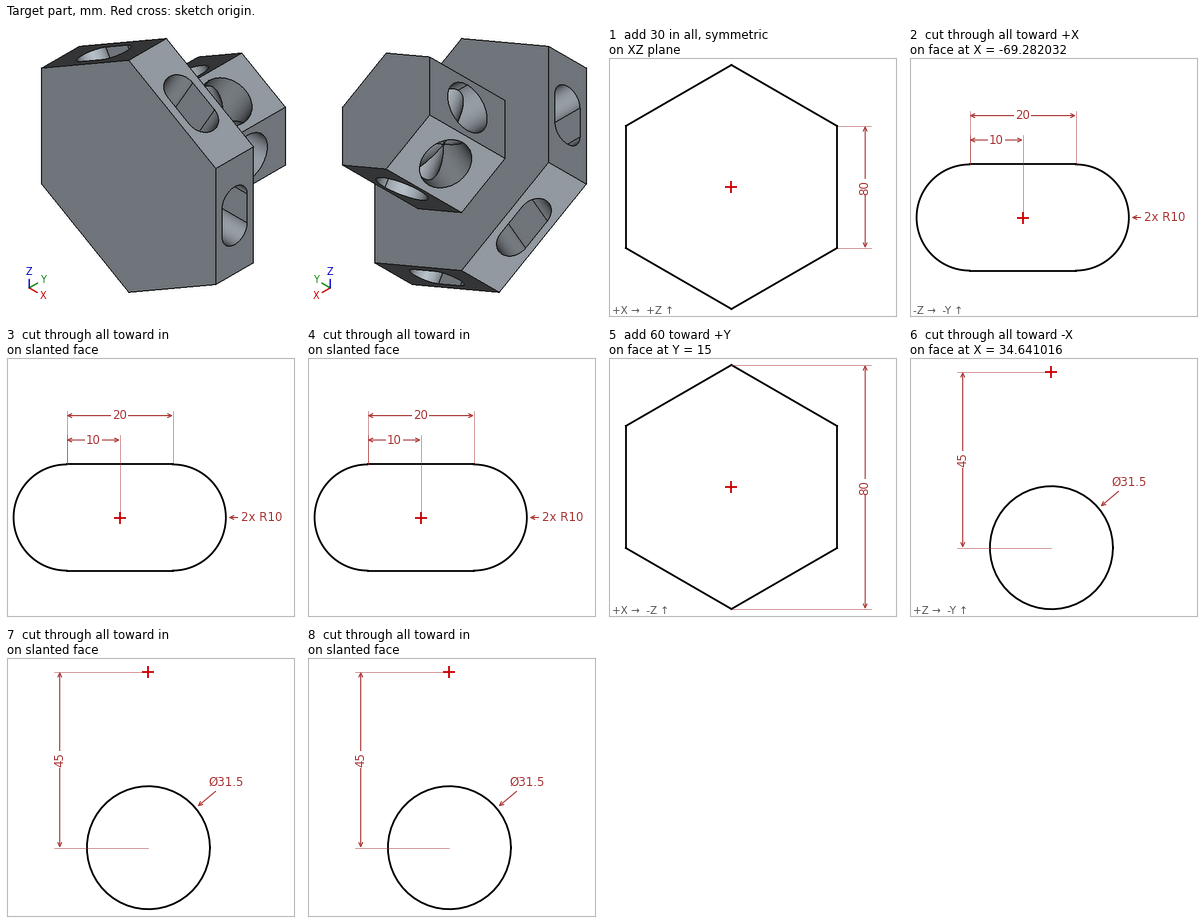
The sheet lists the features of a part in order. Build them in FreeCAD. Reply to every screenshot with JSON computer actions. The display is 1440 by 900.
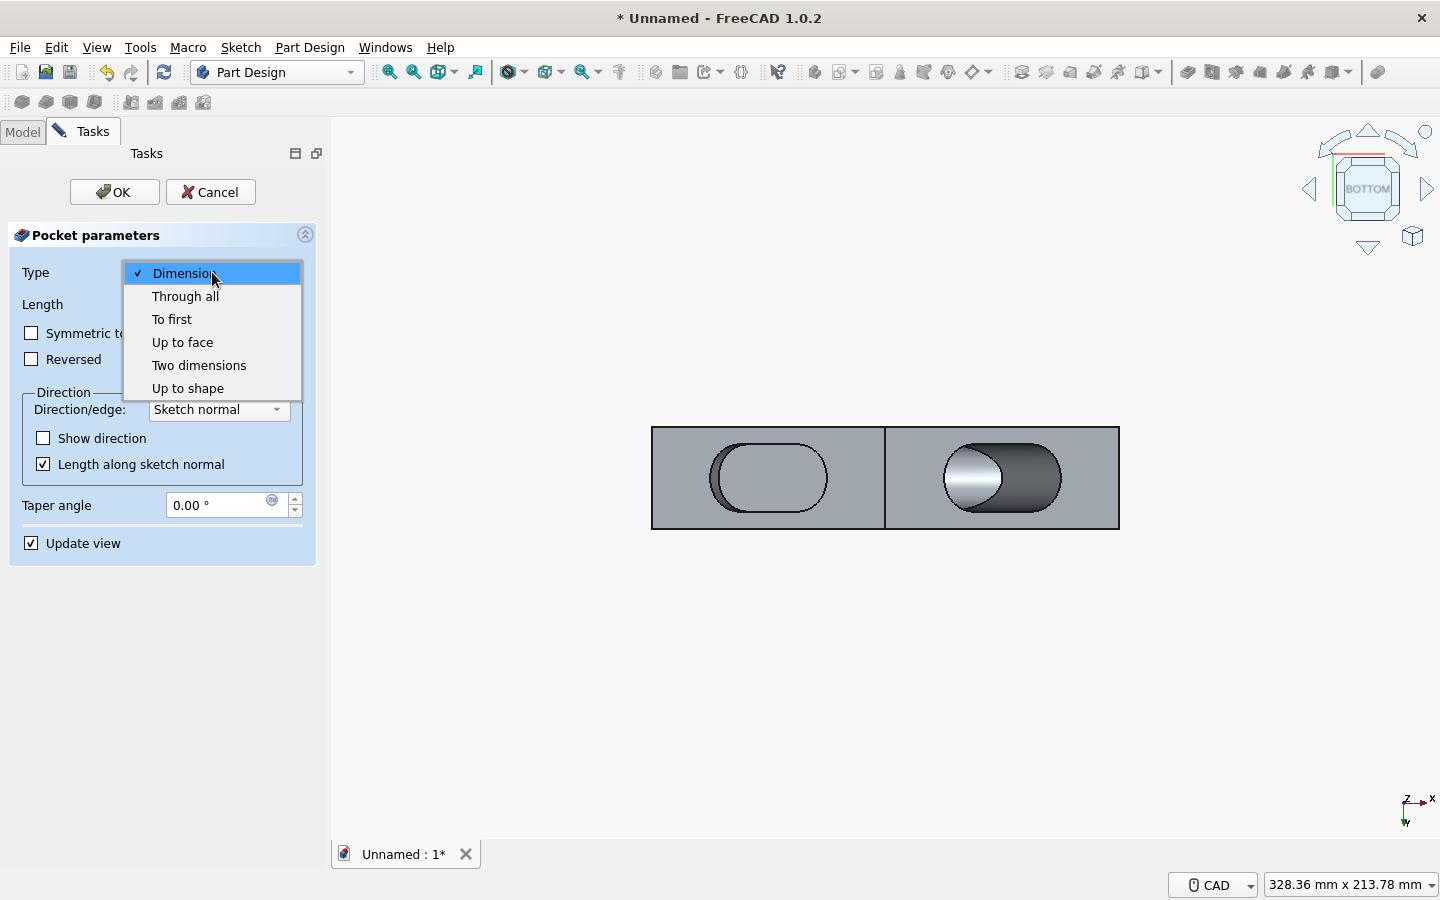
{"action": "left_click", "coordinate": [212, 296]}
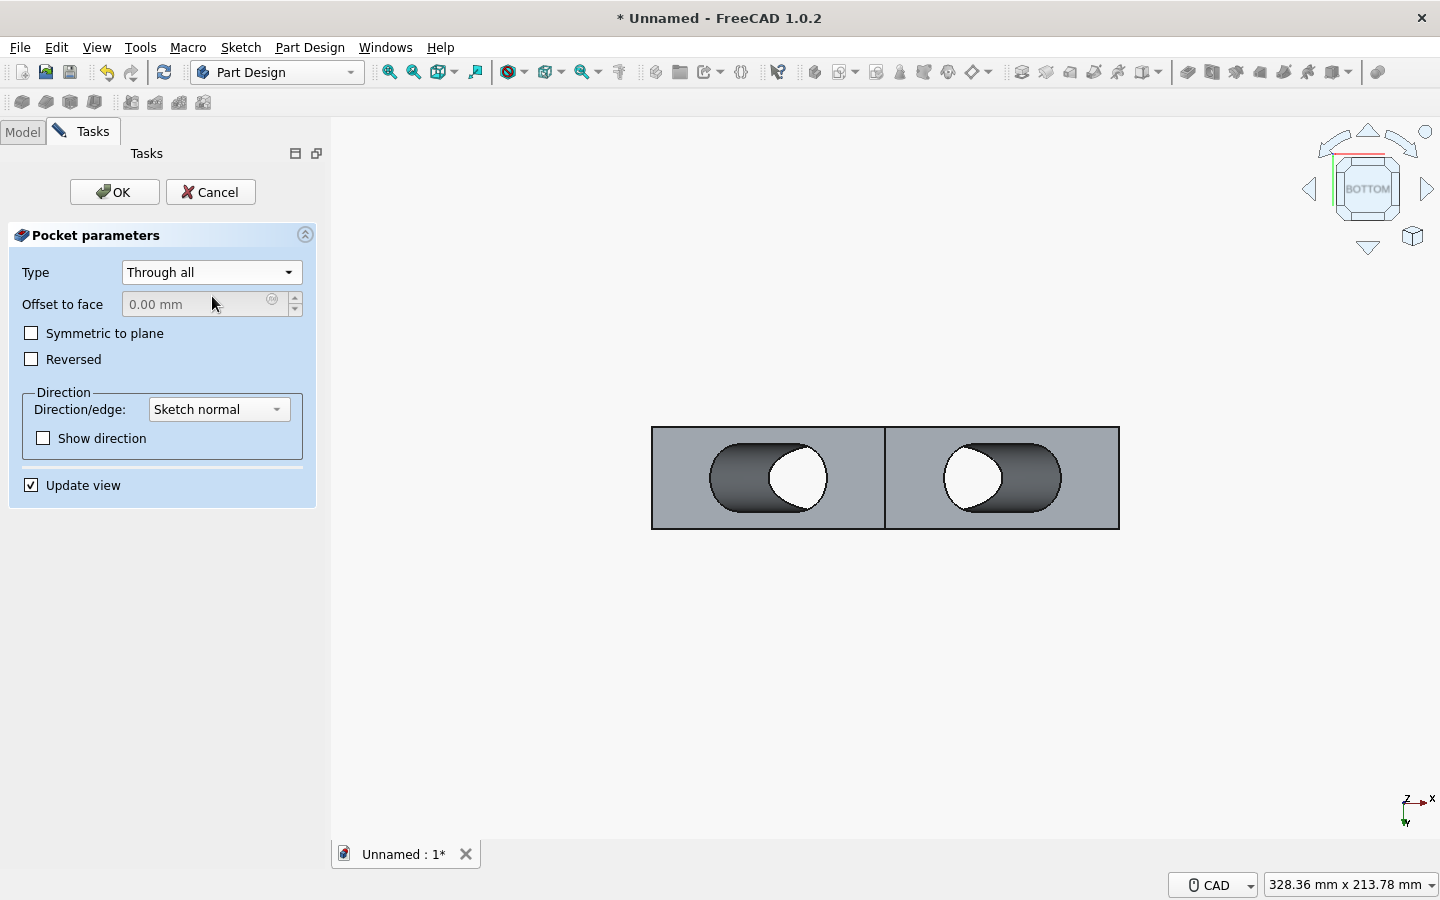
{"action": "left_click", "coordinate": [115, 192]}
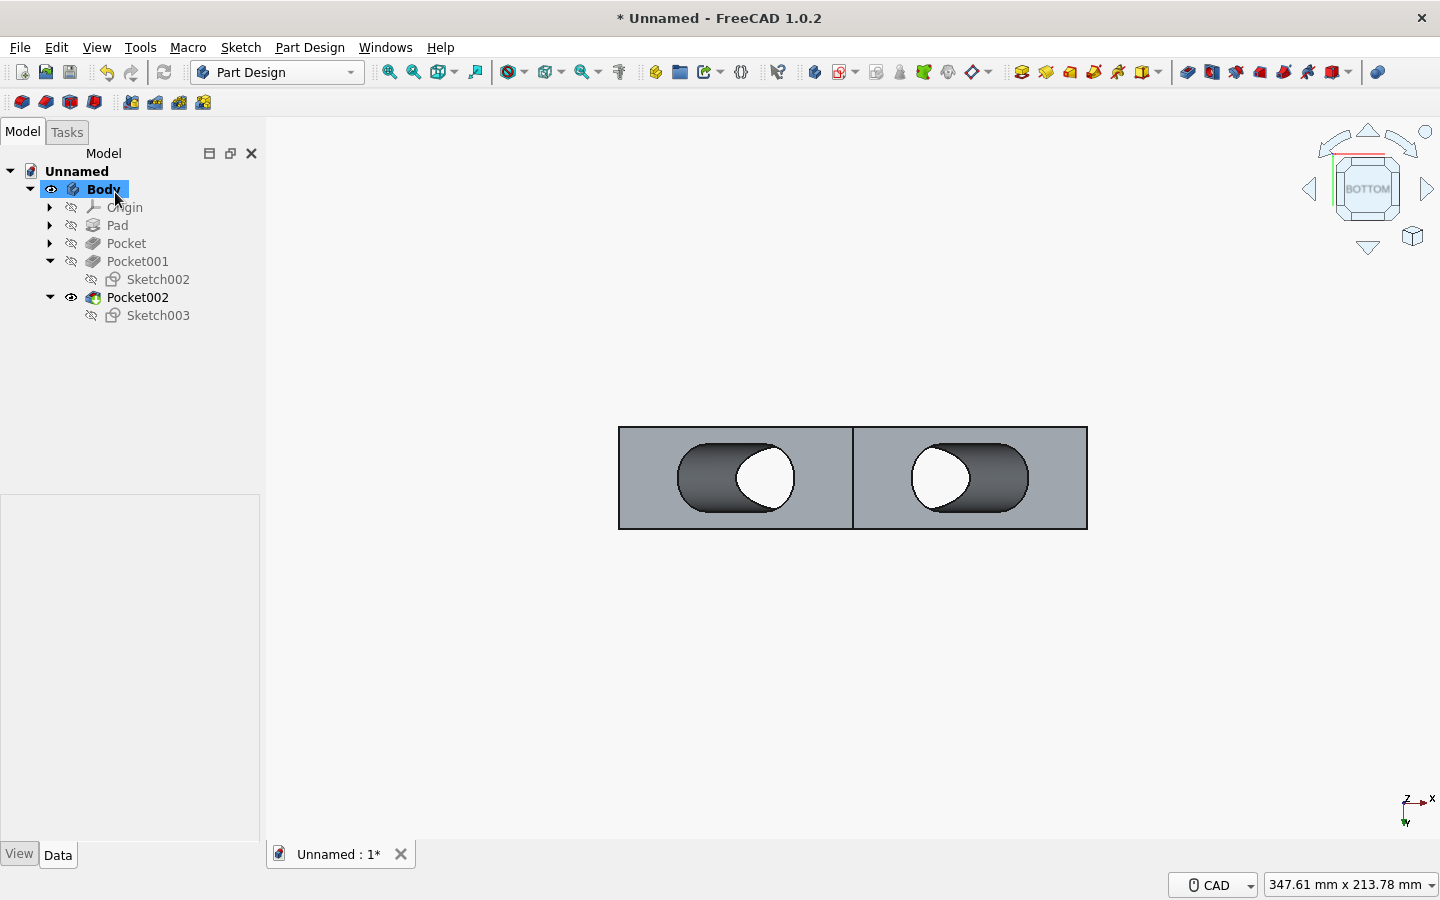
{"action": "left_click", "coordinate": [390, 72]}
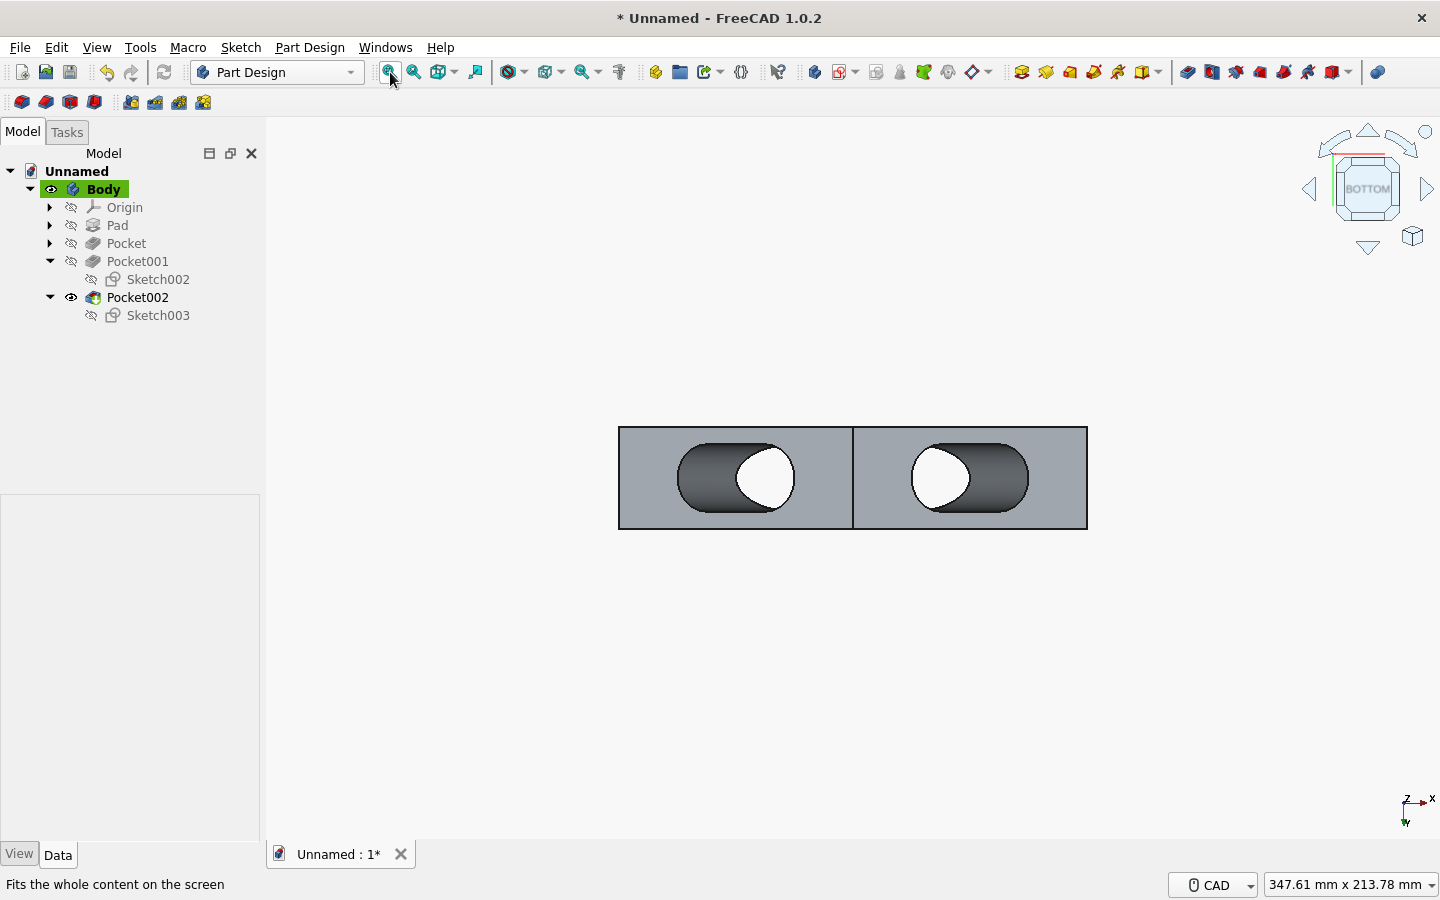
{"action": "key", "text": "4"}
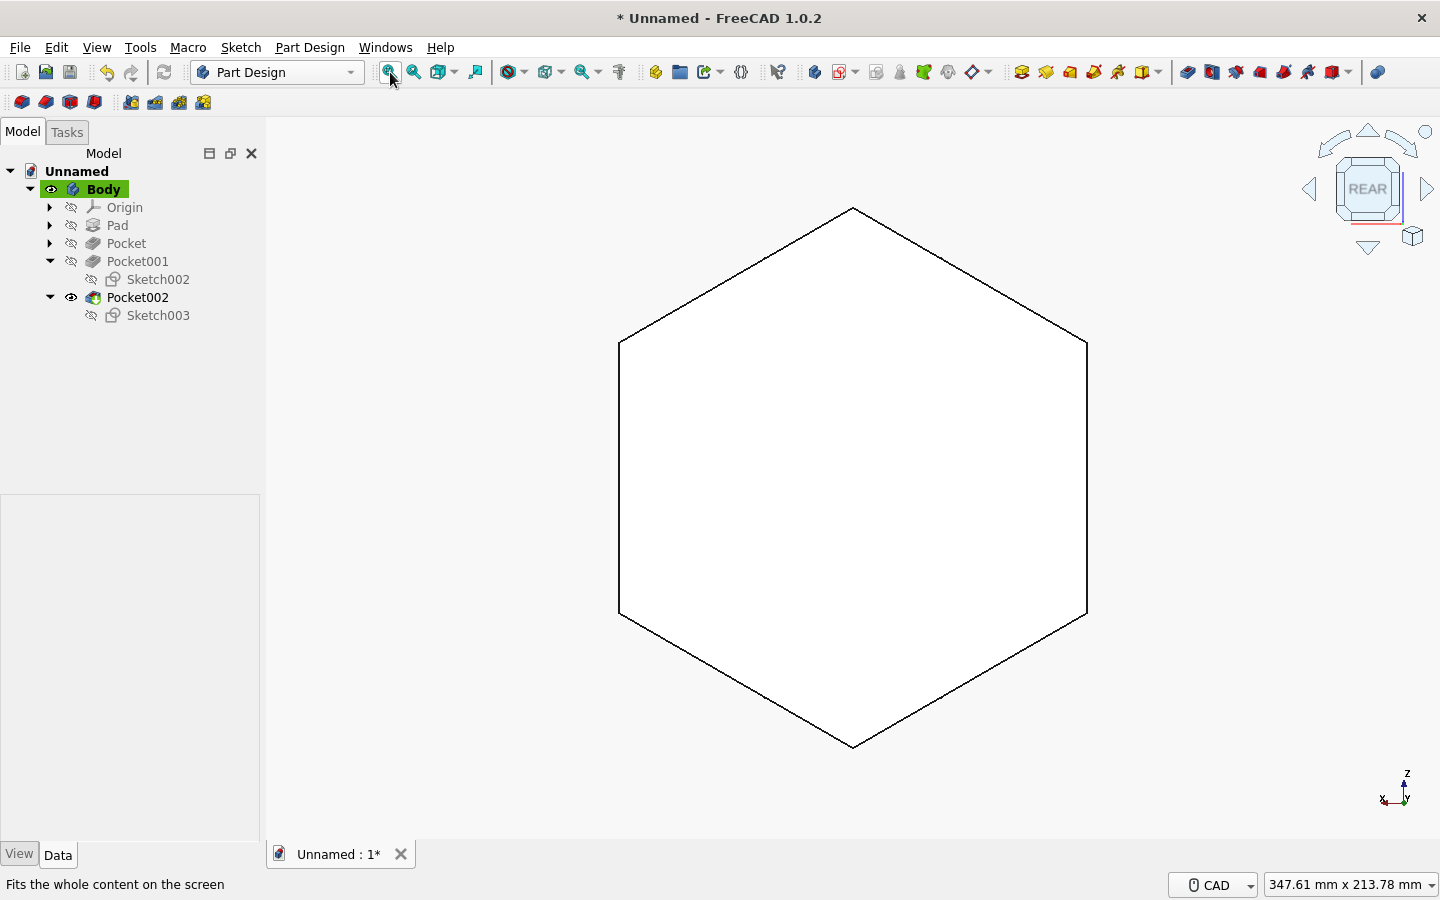
{"action": "left_click", "coordinate": [853, 477]}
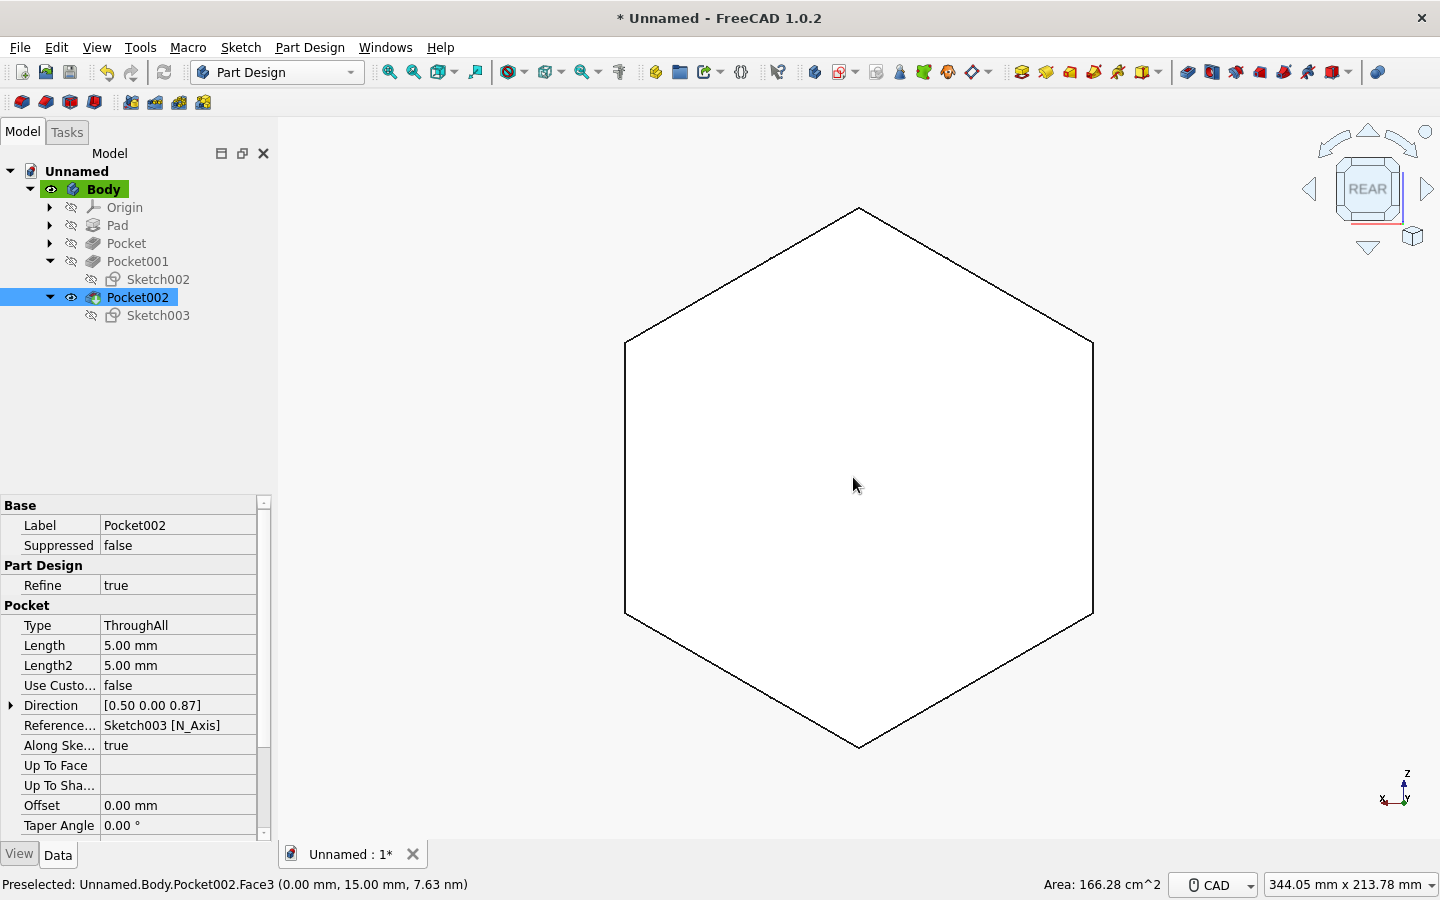
{"action": "left_click", "coordinate": [840, 72]}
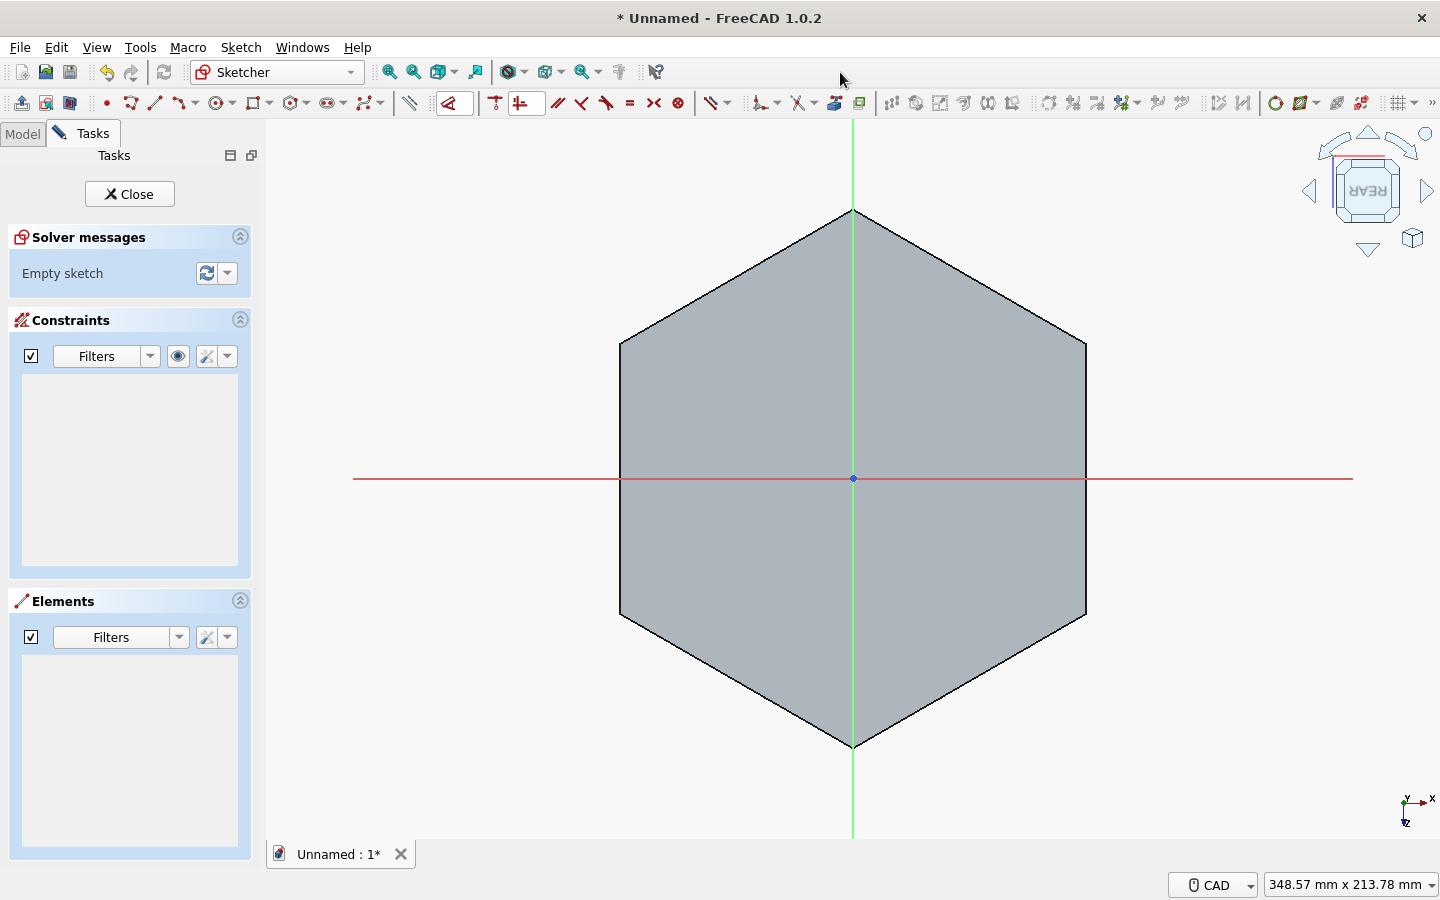
{"action": "scroll", "coordinate": [936, 479], "scroll_direction": "up", "scroll_amount": 3}